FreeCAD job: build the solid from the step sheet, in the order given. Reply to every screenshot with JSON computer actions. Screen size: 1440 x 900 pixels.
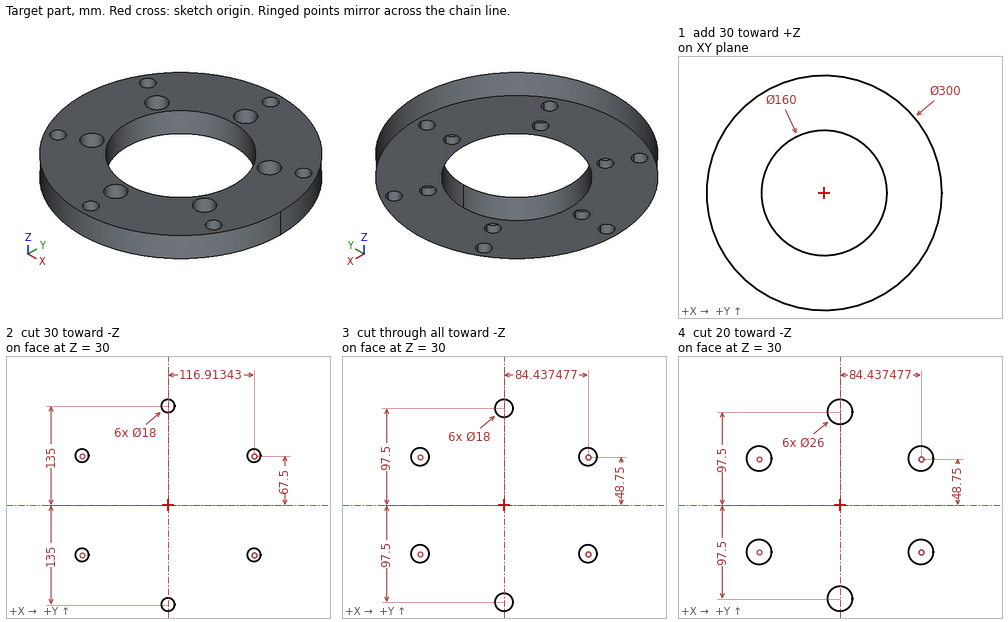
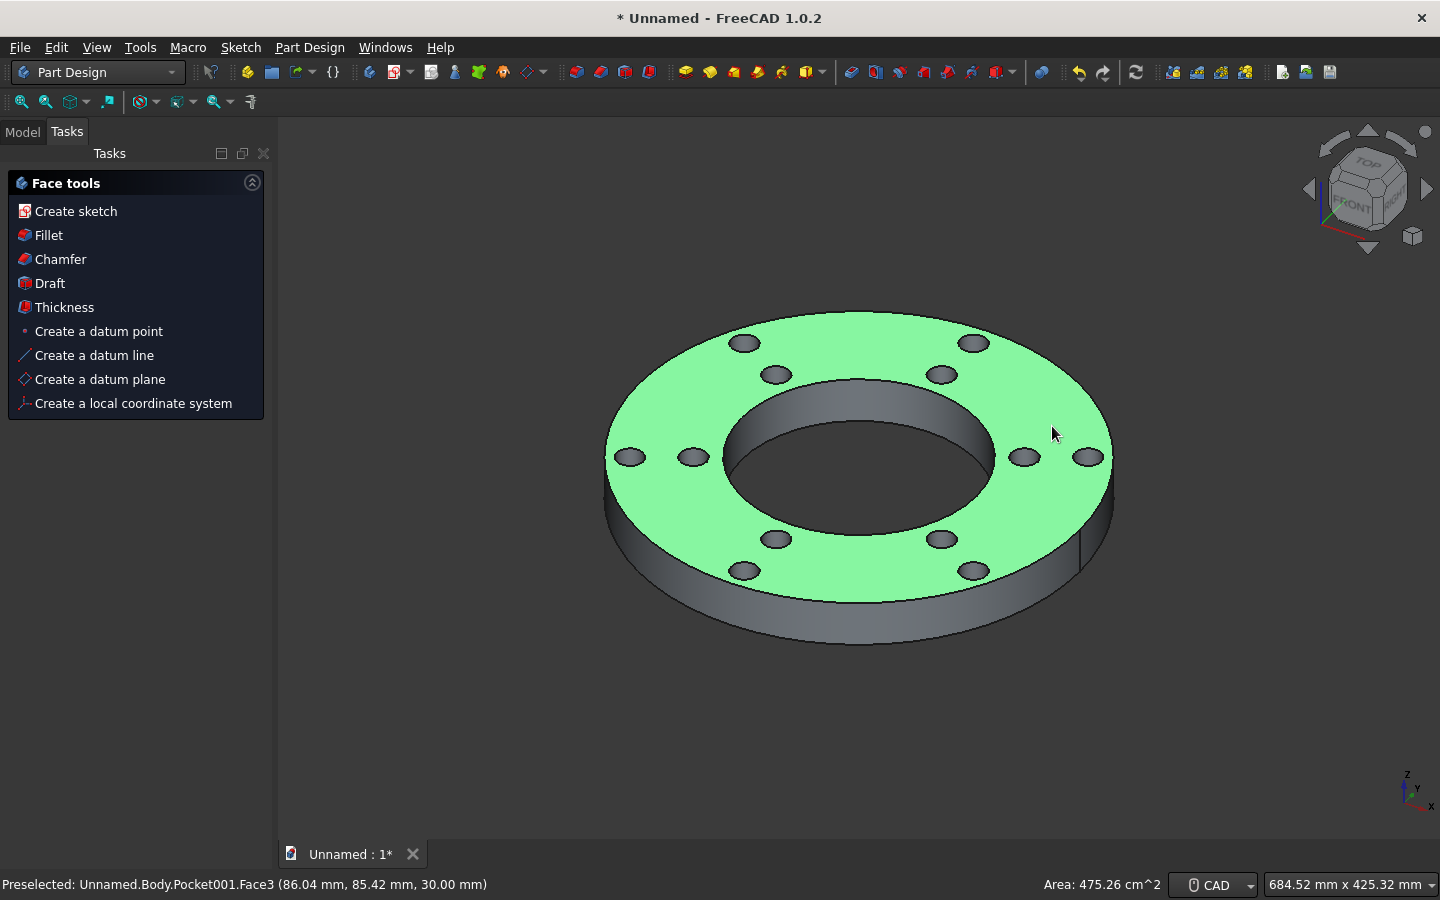
{"action": "left_click", "coordinate": [394, 72]}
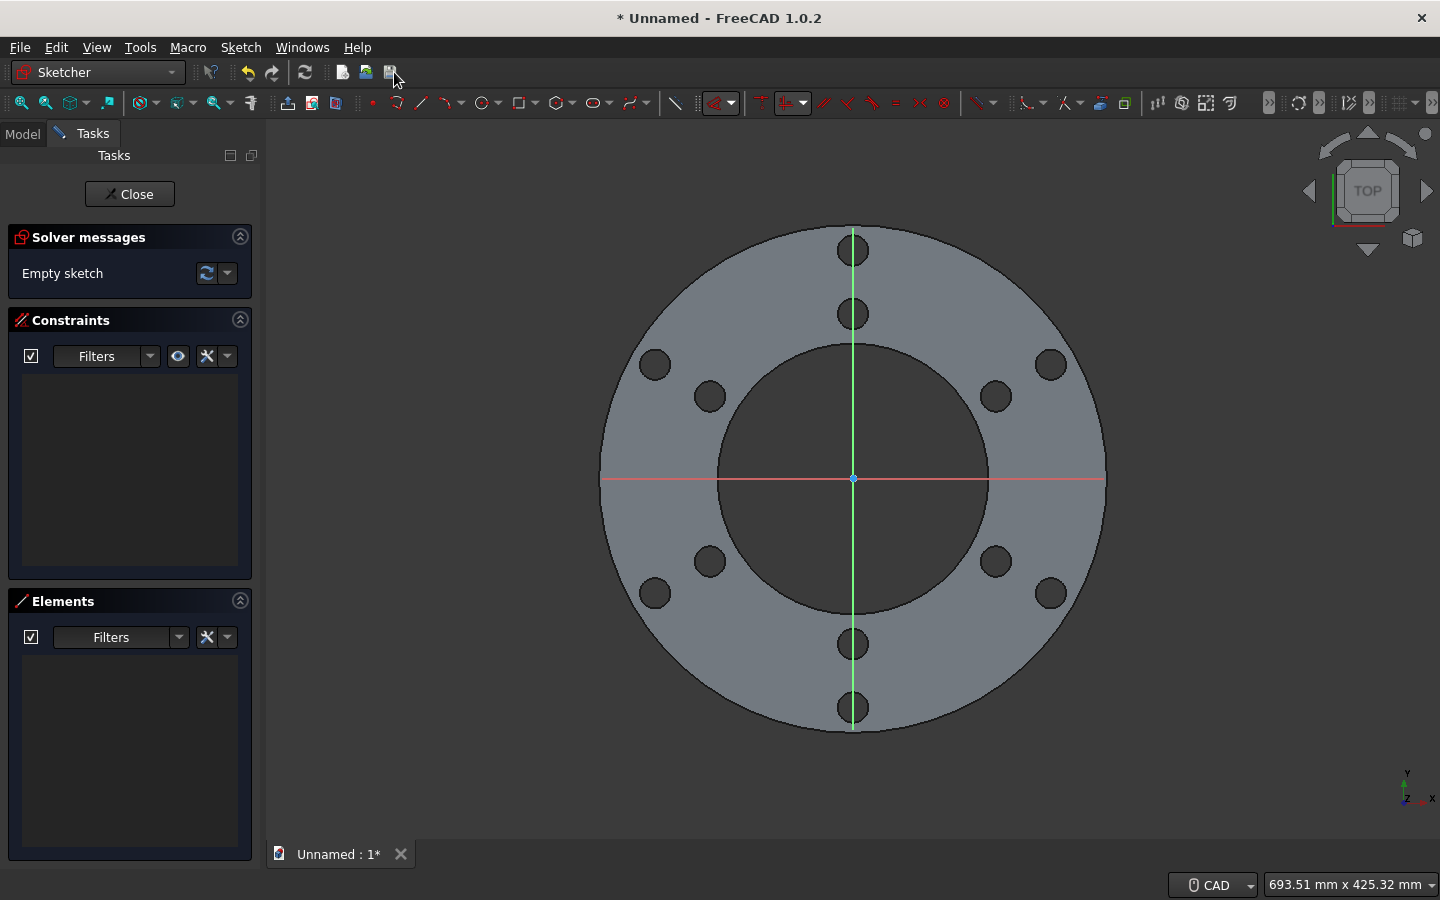
{"action": "left_click", "coordinate": [482, 104]}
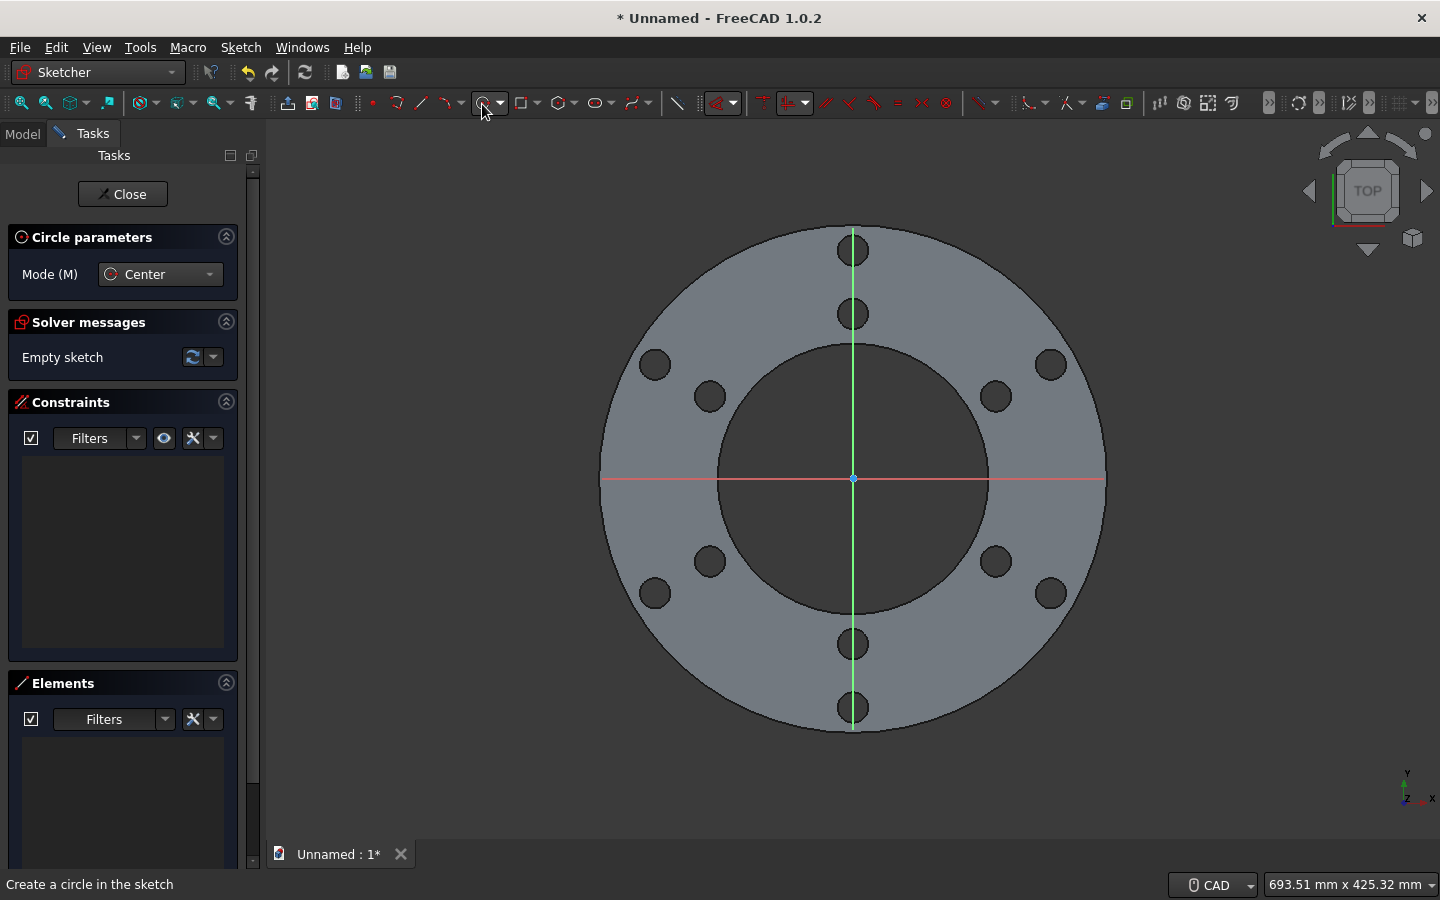
{"action": "left_click", "coordinate": [853, 314]}
{"action": "left_click", "coordinate": [869, 298]}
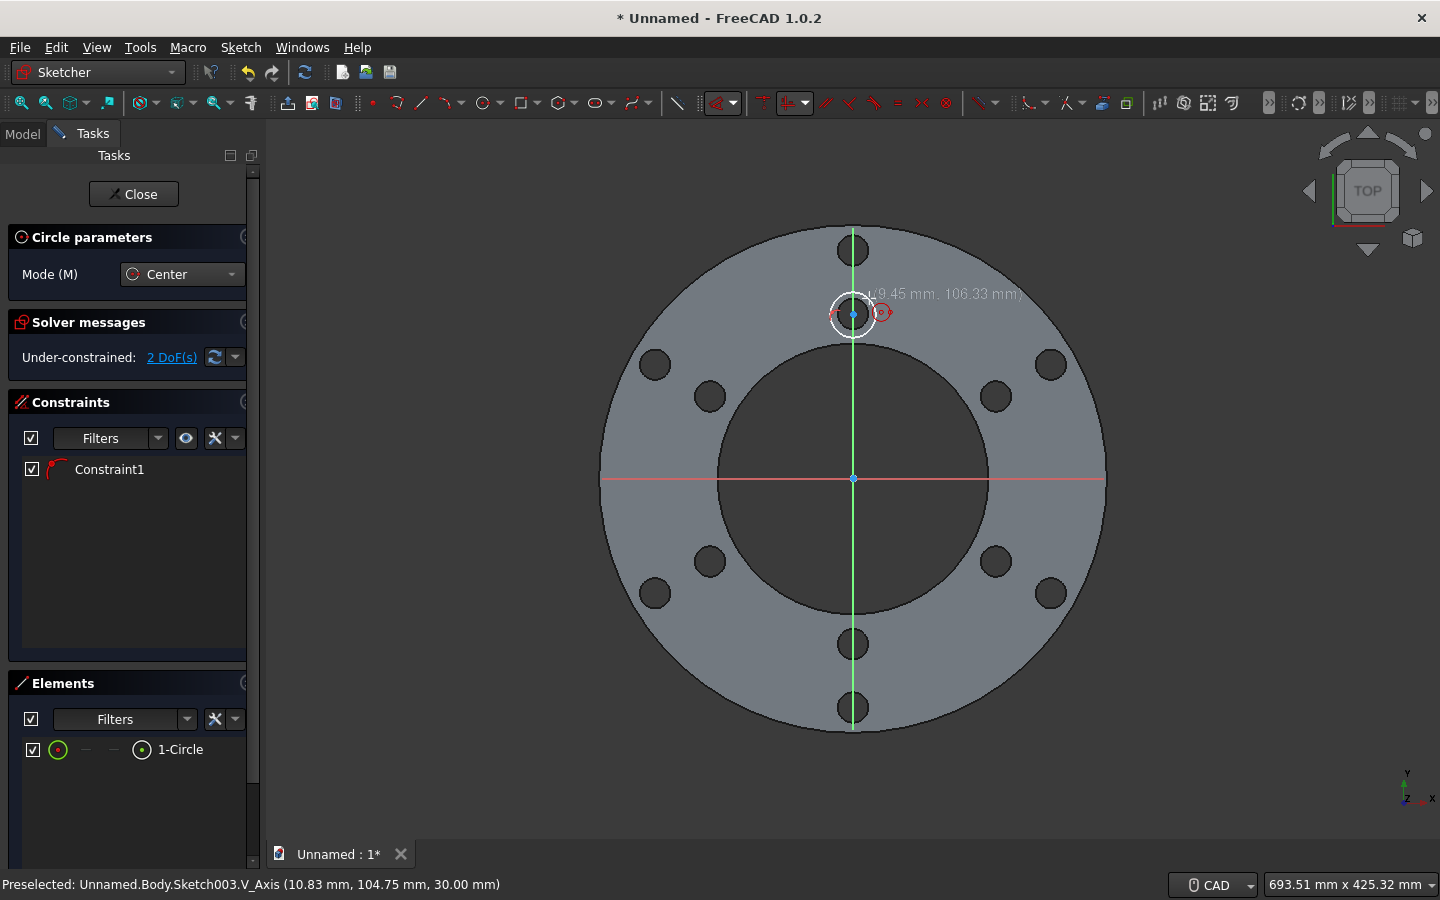
{"action": "left_click", "coordinate": [996, 396]}
{"action": "left_click", "coordinate": [1011, 381]}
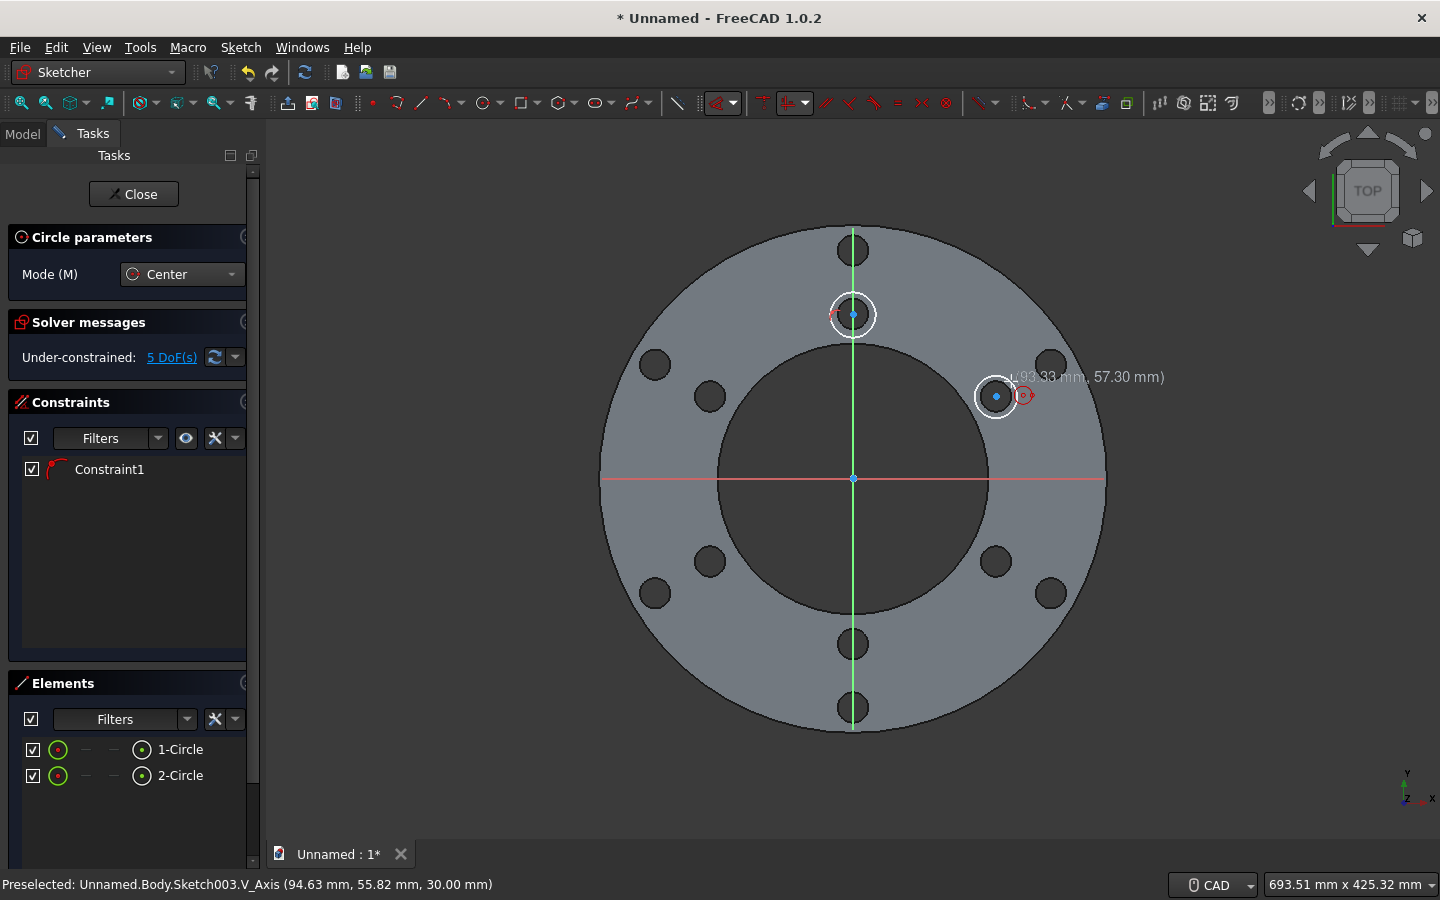
{"action": "left_click", "coordinate": [996, 562]}
{"action": "left_click", "coordinate": [1011, 546]}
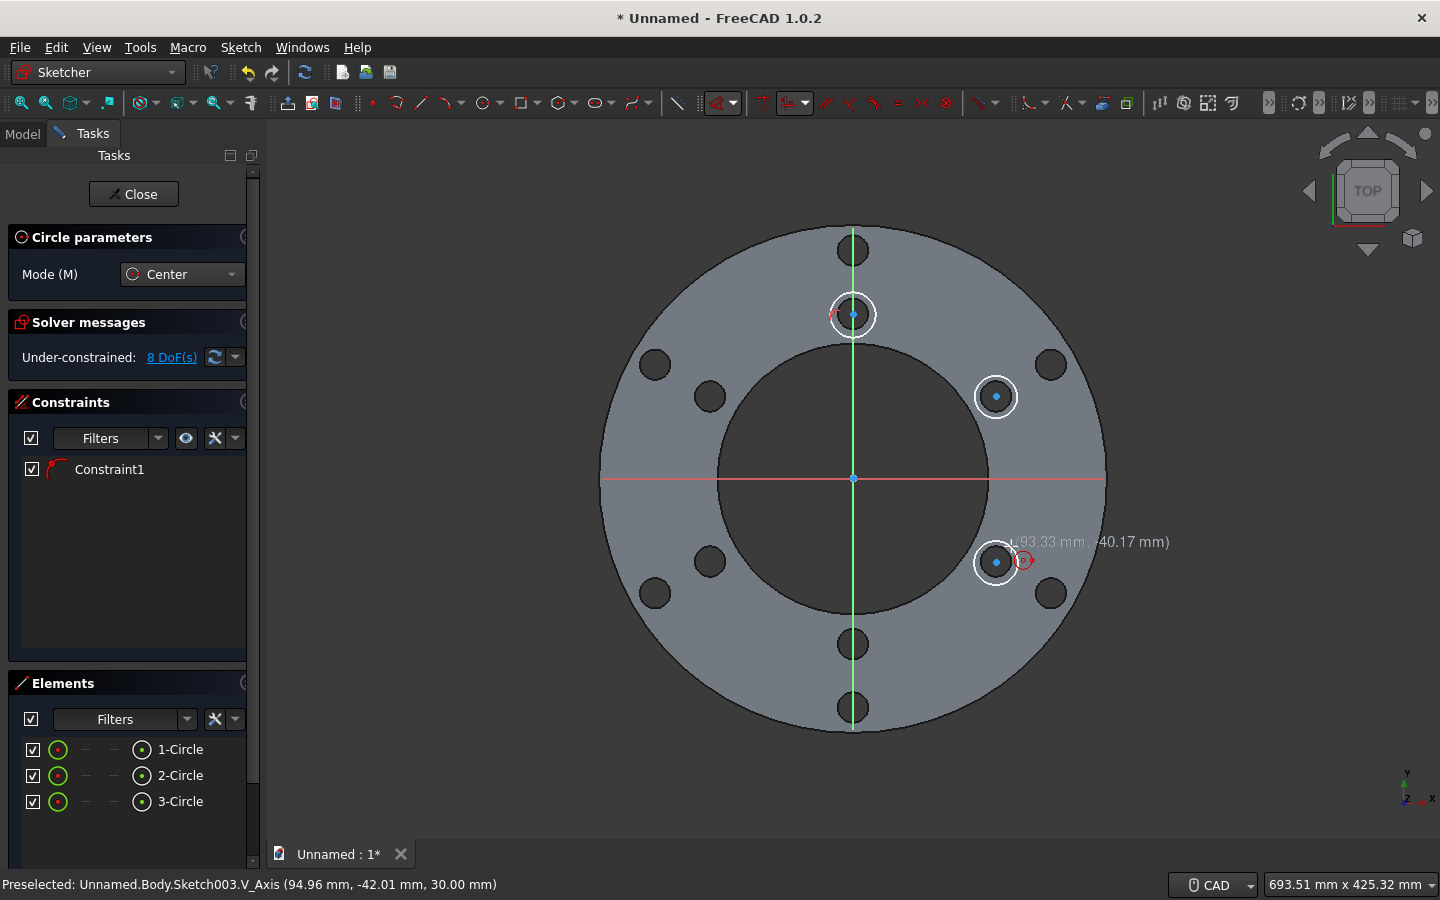
{"action": "left_click", "coordinate": [853, 644]}
{"action": "left_click", "coordinate": [869, 628]}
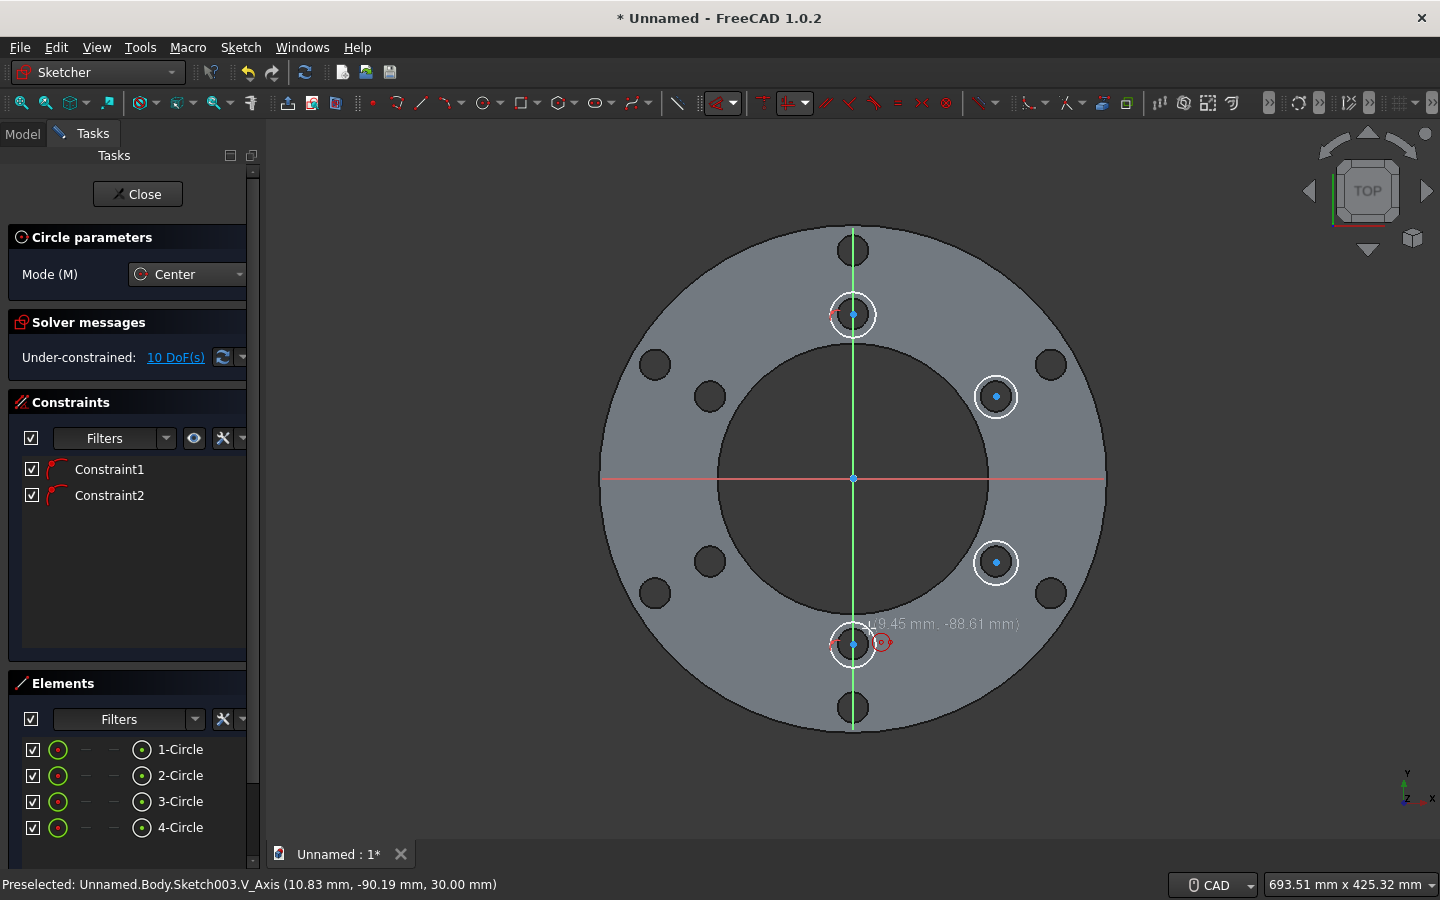
{"action": "left_click", "coordinate": [710, 562]}
{"action": "left_click", "coordinate": [726, 546]}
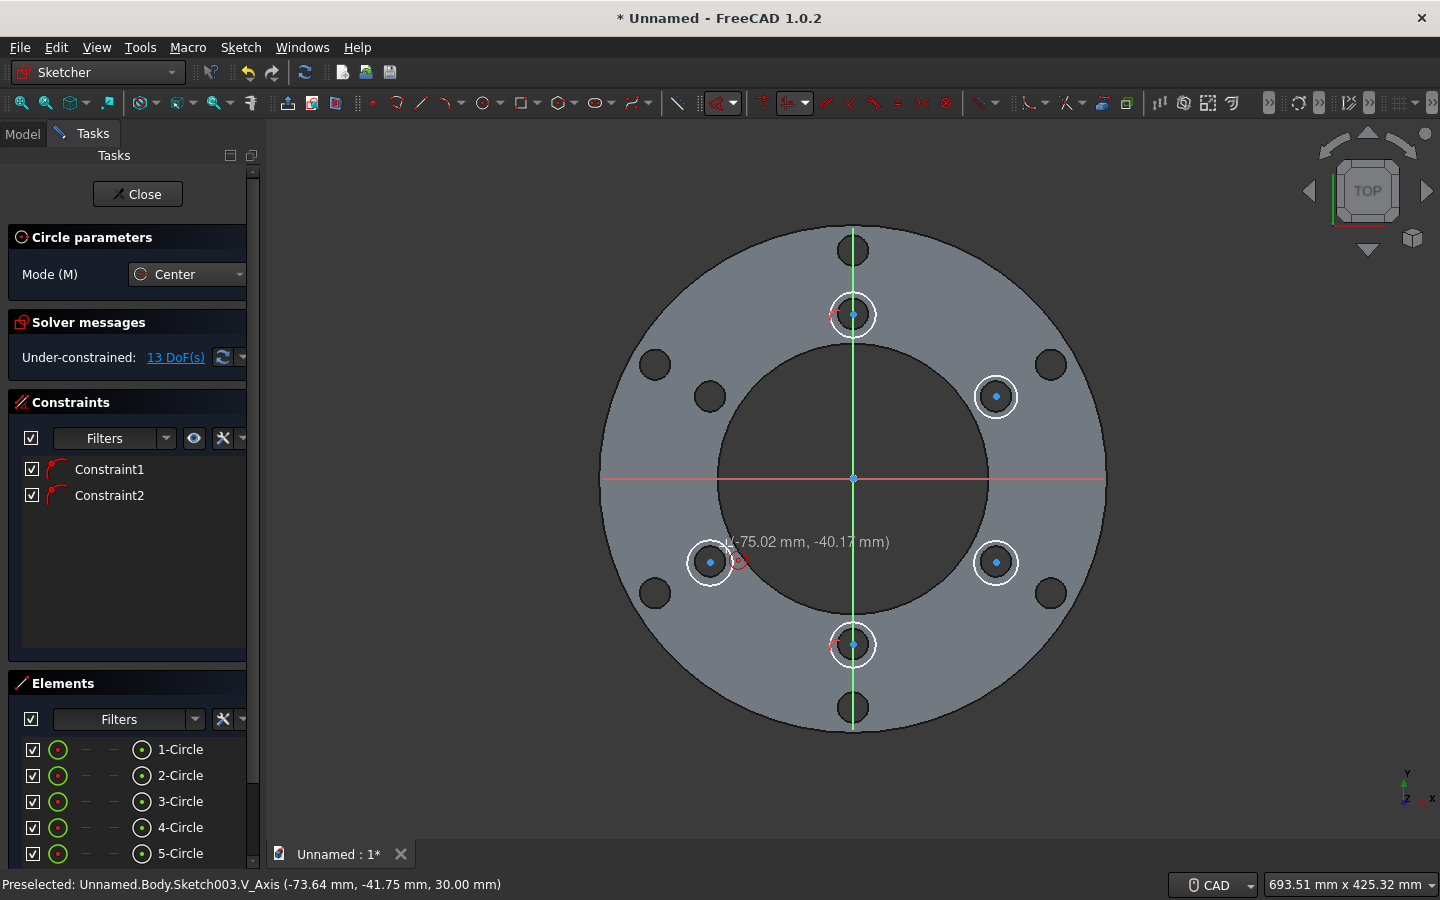
{"action": "left_click", "coordinate": [710, 396]}
{"action": "left_click", "coordinate": [726, 381]}
{"action": "key", "text": "Escape"}